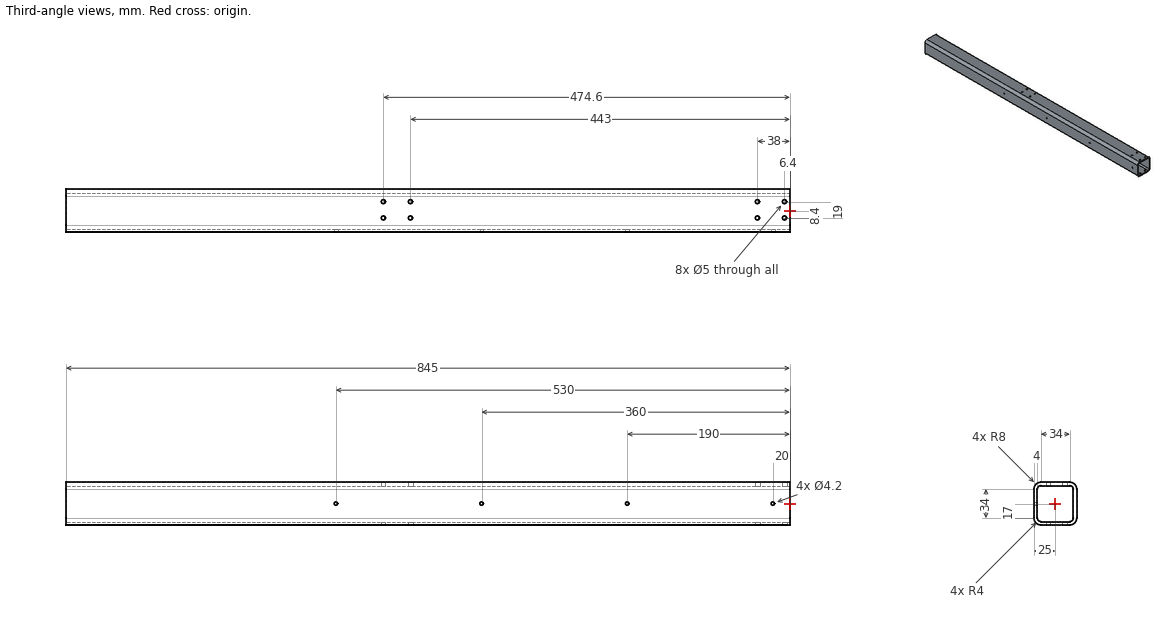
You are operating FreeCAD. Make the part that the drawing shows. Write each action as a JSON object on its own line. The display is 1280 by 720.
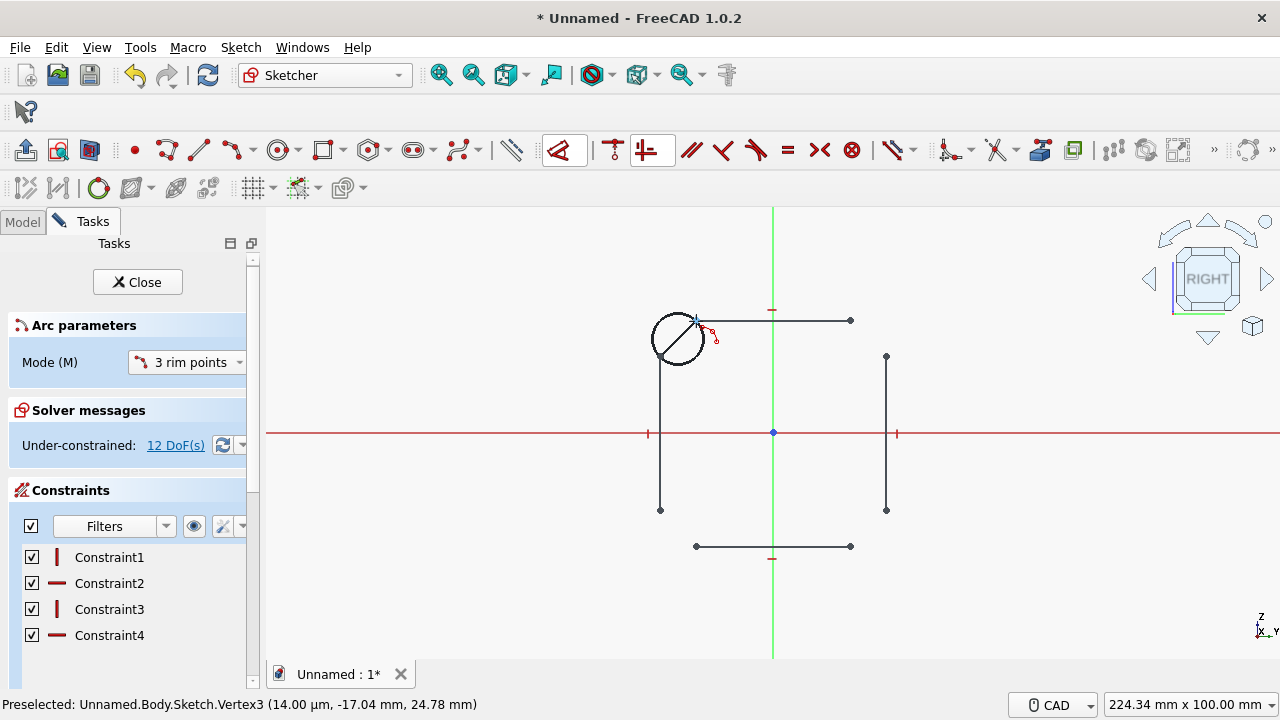
{"action": "scroll", "coordinate": [671, 331], "scroll_direction": "up", "scroll_amount": 3}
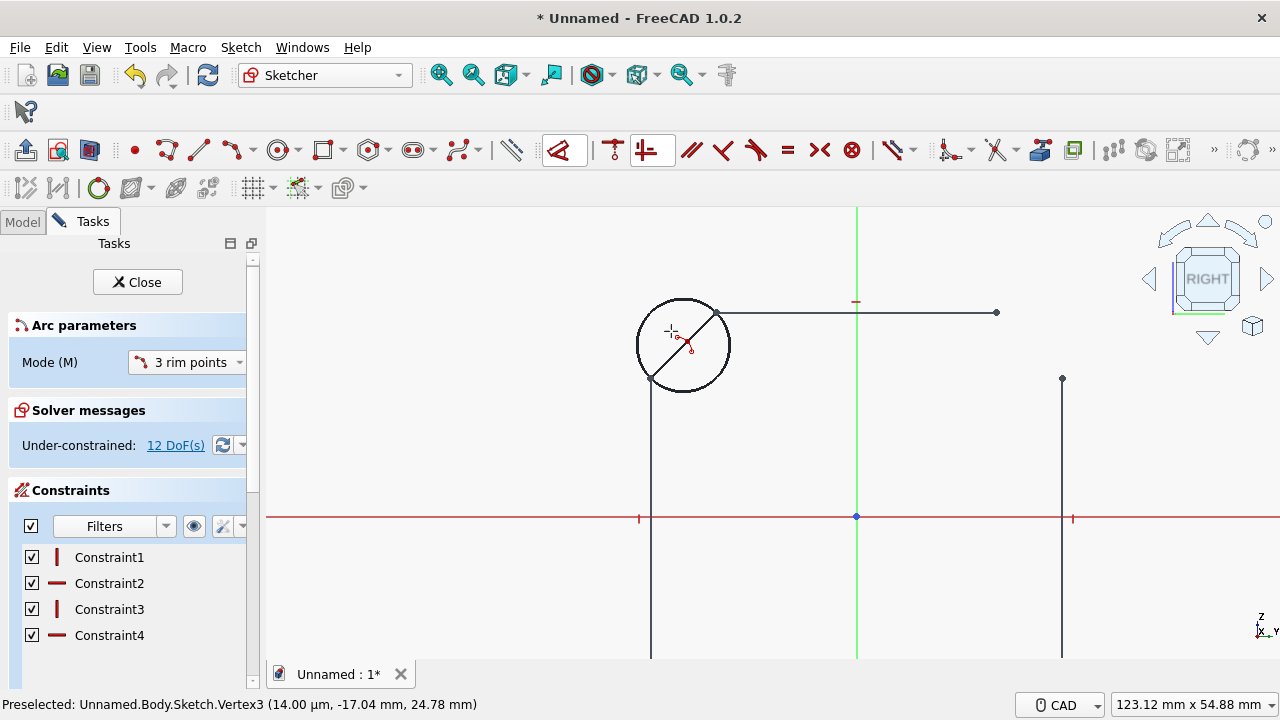
{"action": "left_click", "coordinate": [670, 330]}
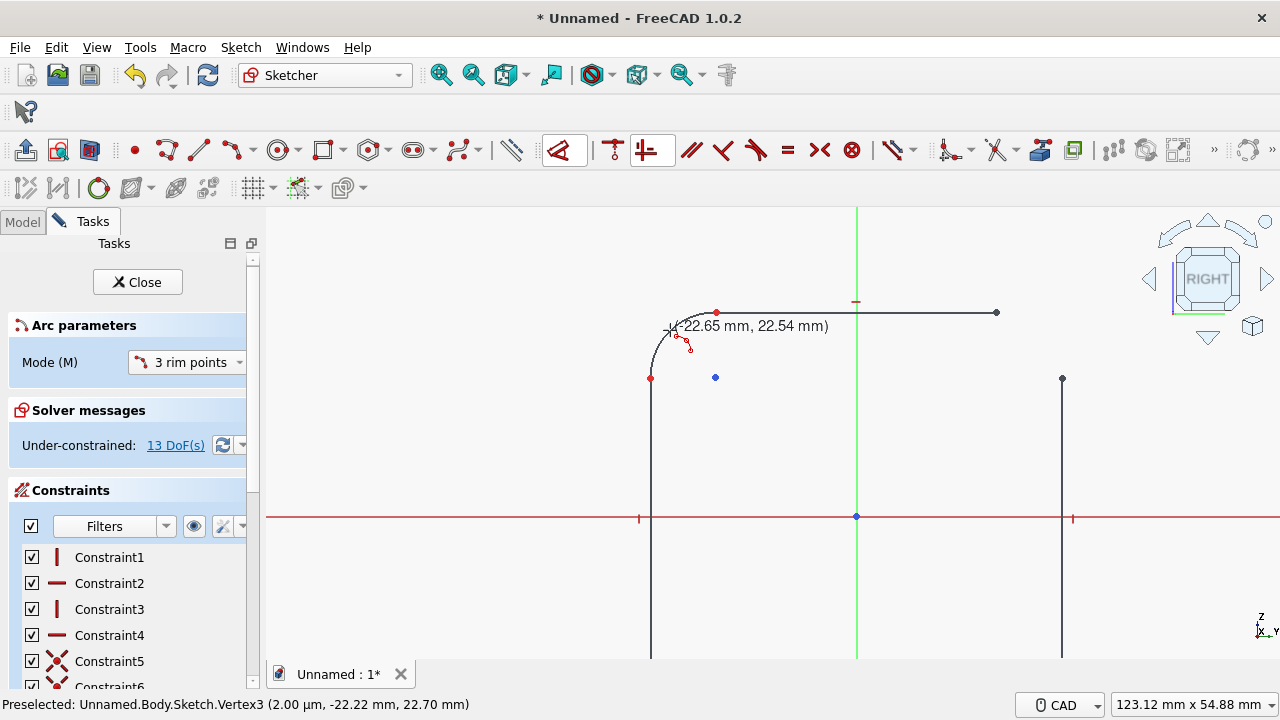
{"action": "left_click", "coordinate": [997, 313]}
{"action": "left_click", "coordinate": [1062, 378]}
{"action": "left_click", "coordinate": [1043, 330]}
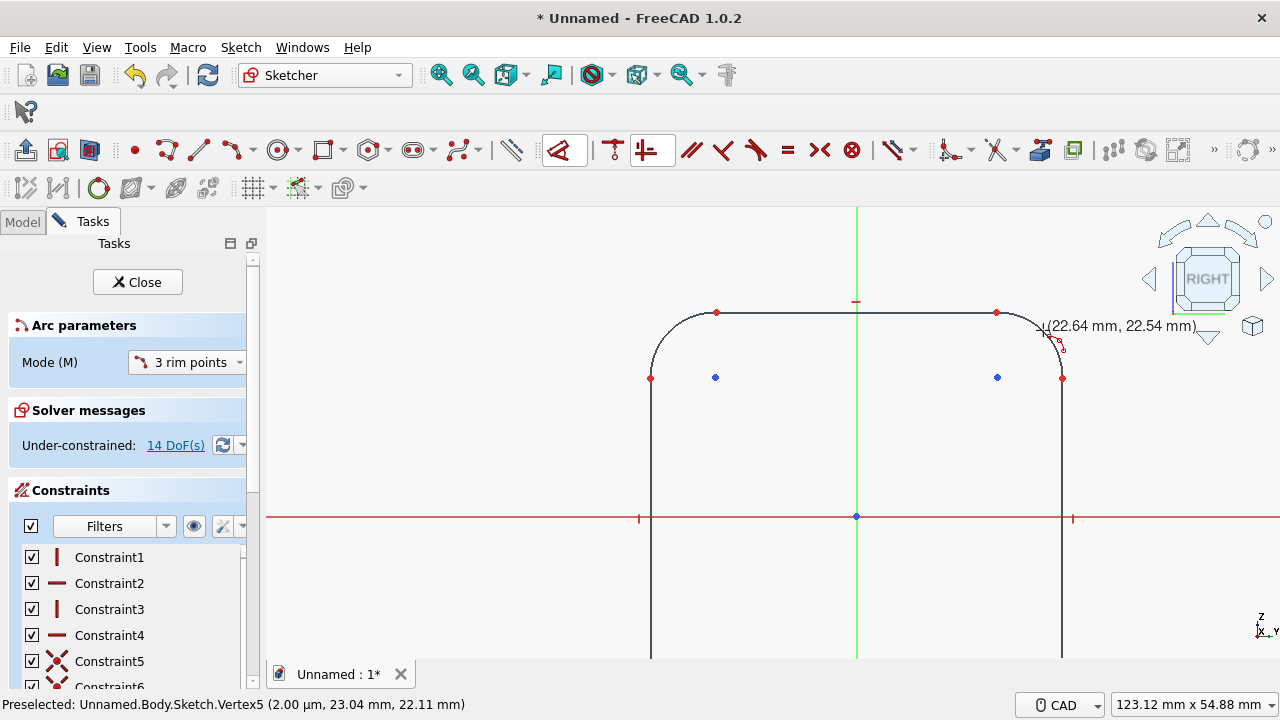
{"action": "scroll", "coordinate": [395, 263], "scroll_direction": "down", "scroll_amount": 2}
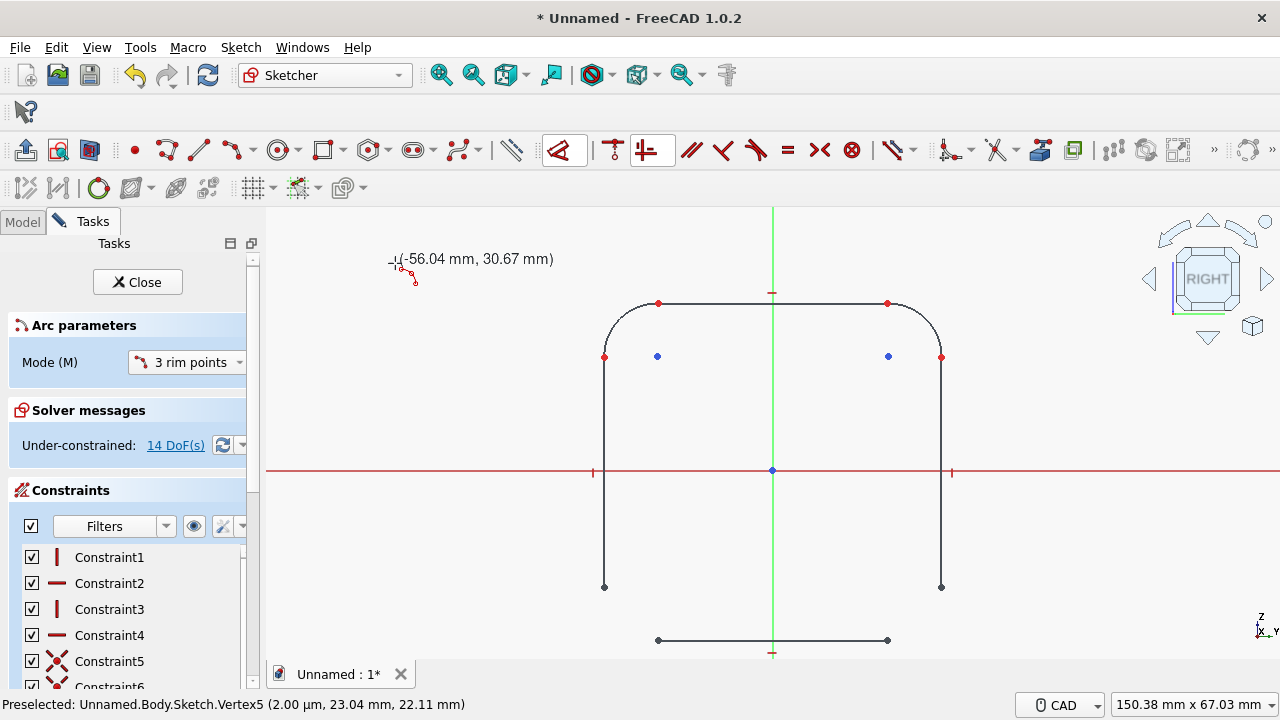
{"action": "left_click", "coordinate": [842, 528]}
{"action": "left_click", "coordinate": [798, 572]}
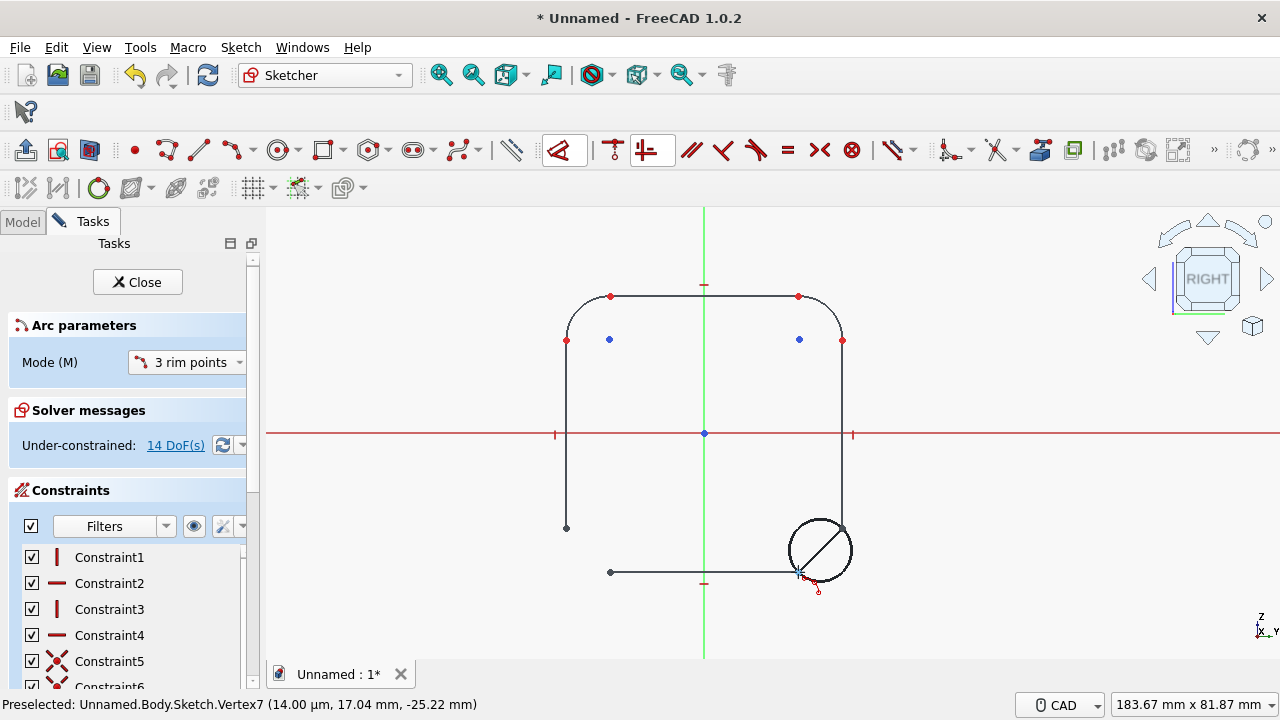
{"action": "scroll", "coordinate": [829, 558], "scroll_direction": "up", "scroll_amount": 2}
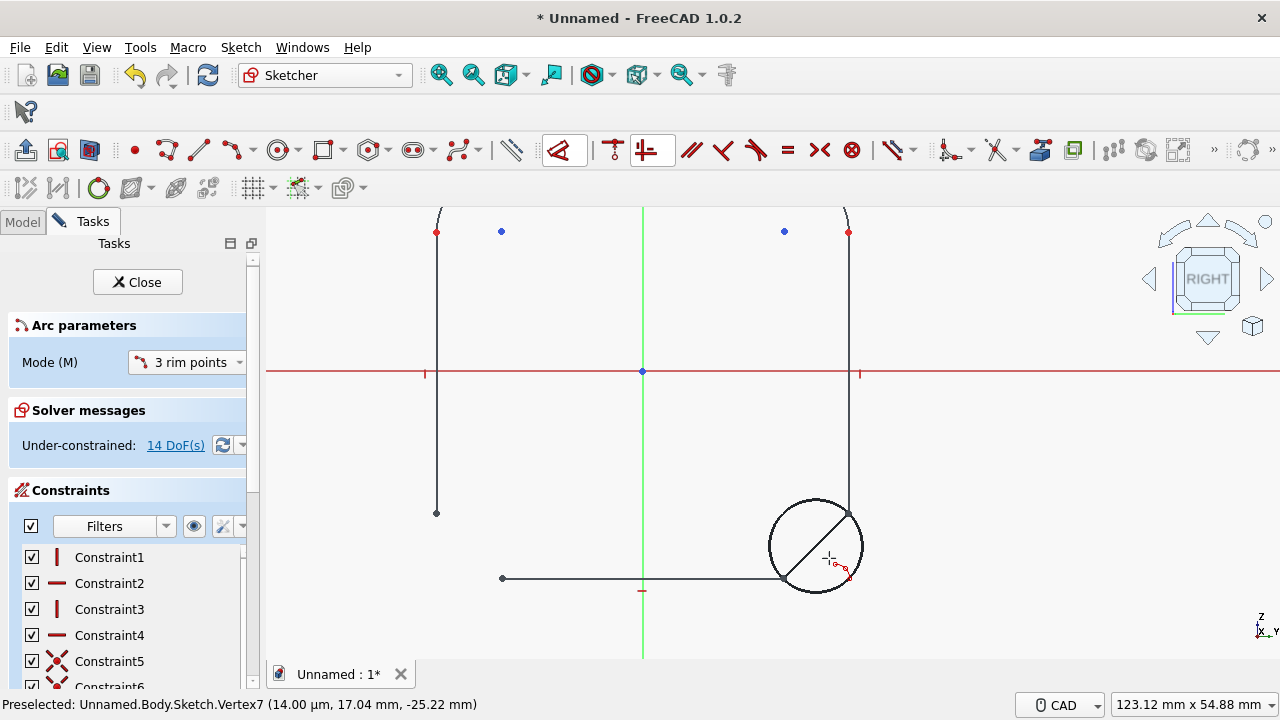
{"action": "left_click", "coordinate": [829, 558]}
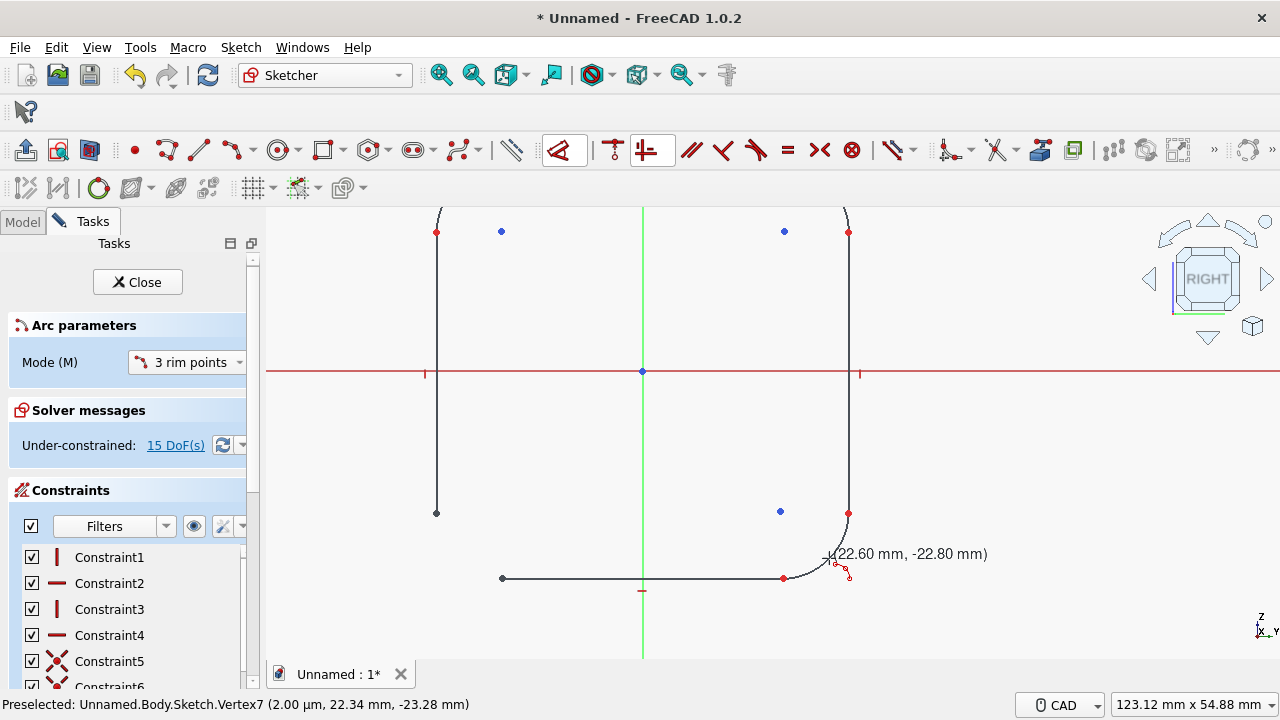
{"action": "left_click", "coordinate": [503, 579]}
{"action": "left_click", "coordinate": [437, 513]}
{"action": "left_click", "coordinate": [456, 558]}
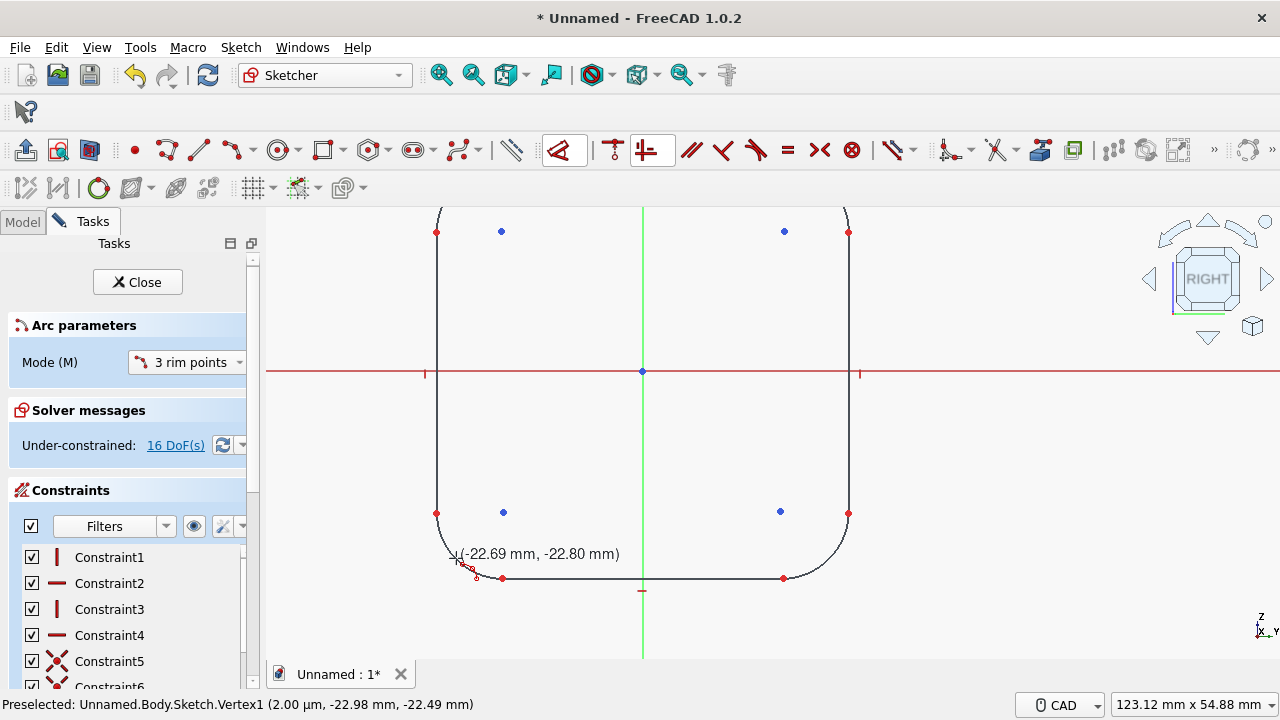
{"action": "left_click", "coordinate": [200, 150]}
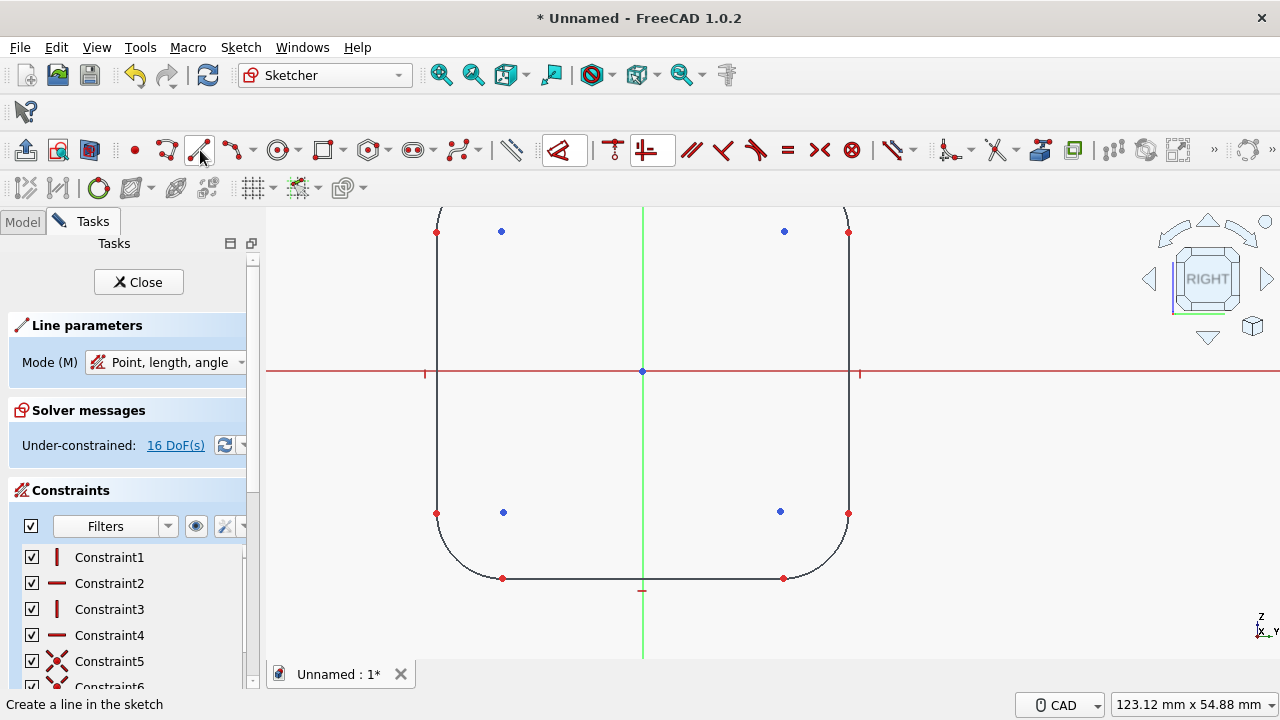
{"action": "scroll", "coordinate": [830, 559], "scroll_direction": "down", "scroll_amount": 2}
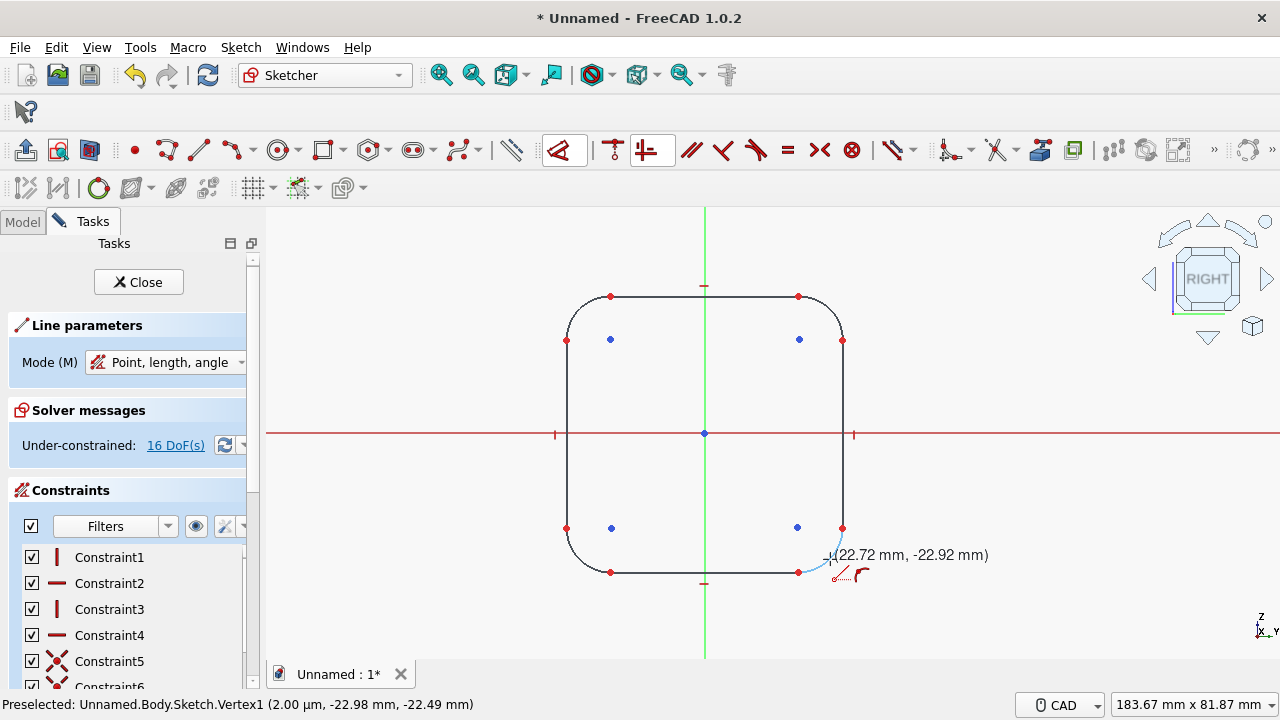
{"action": "left_click", "coordinate": [589, 340]}
{"action": "left_click", "coordinate": [589, 527]}